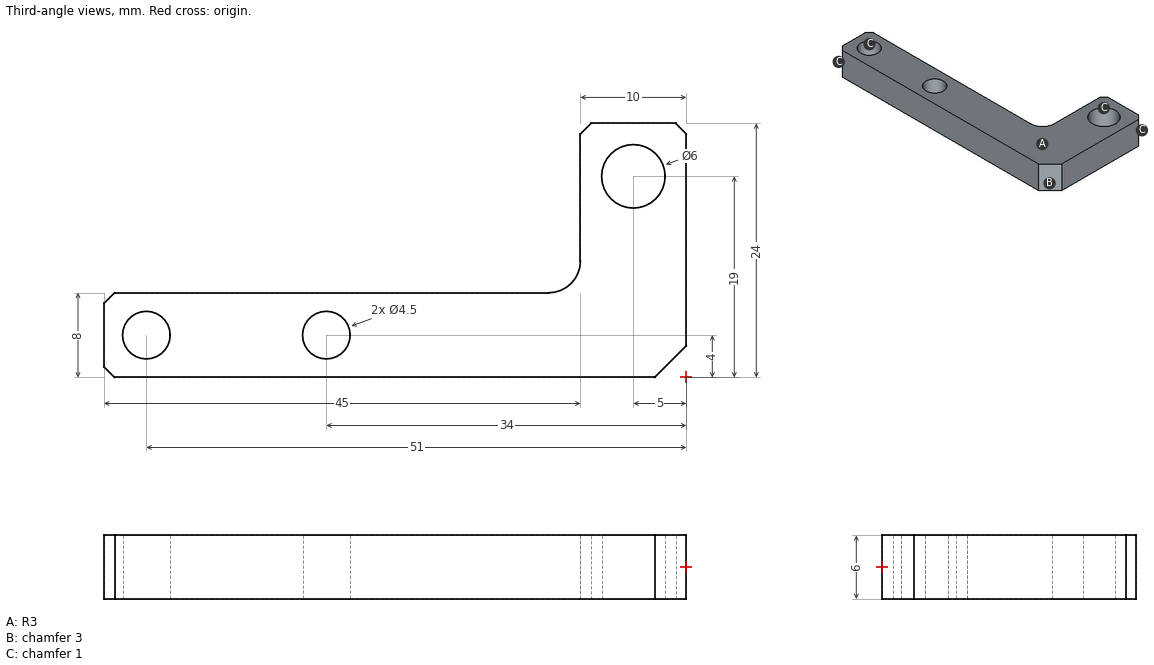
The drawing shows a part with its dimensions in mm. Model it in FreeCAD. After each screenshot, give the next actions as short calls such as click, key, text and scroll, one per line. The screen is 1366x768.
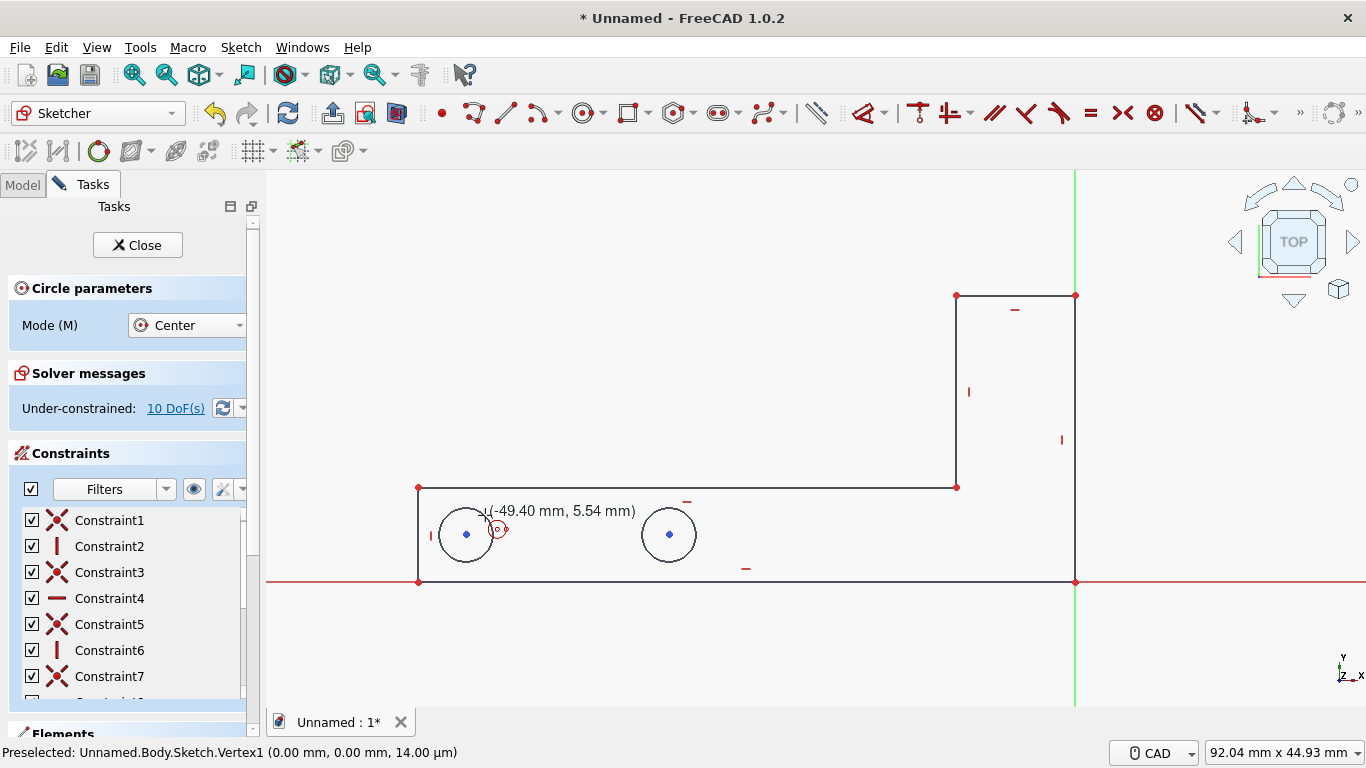
click(1016, 355)
click(1041, 330)
key(Escape)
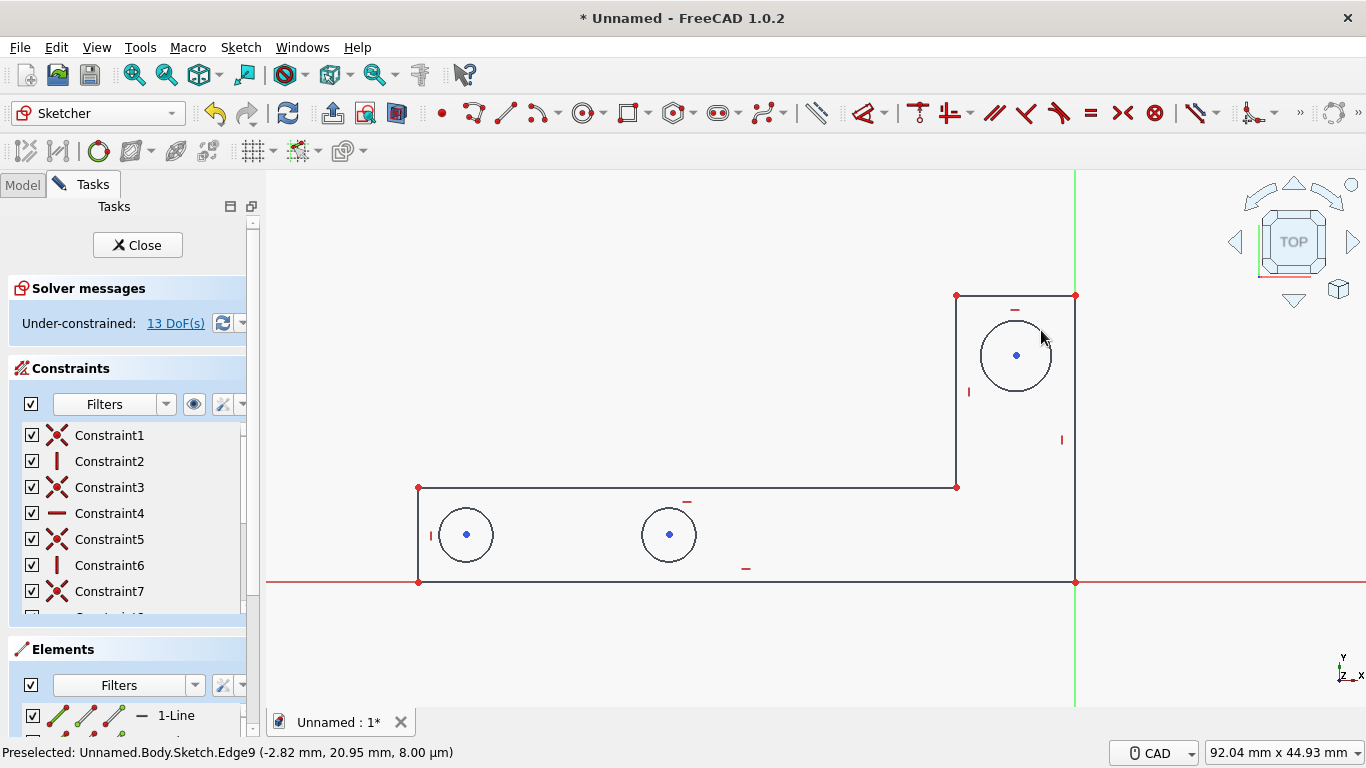
click(688, 516)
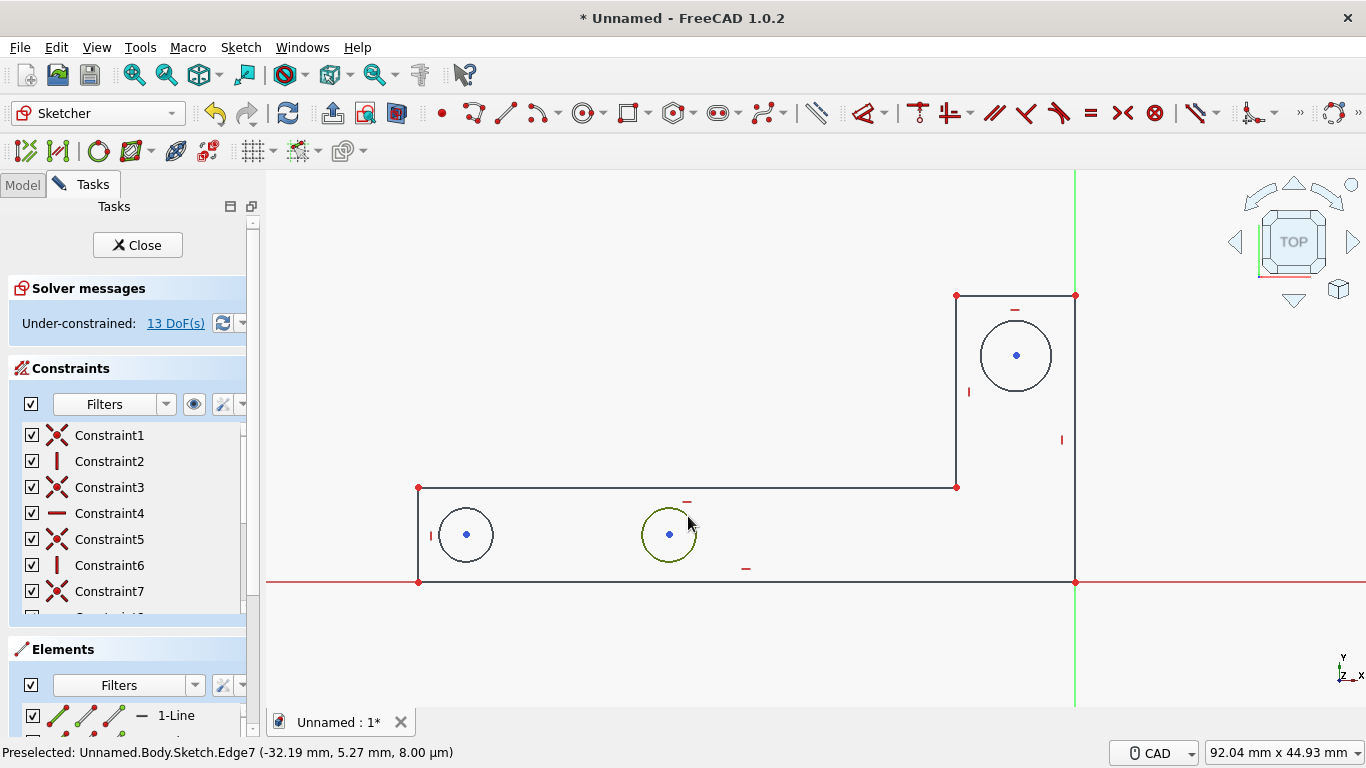
click(485, 516)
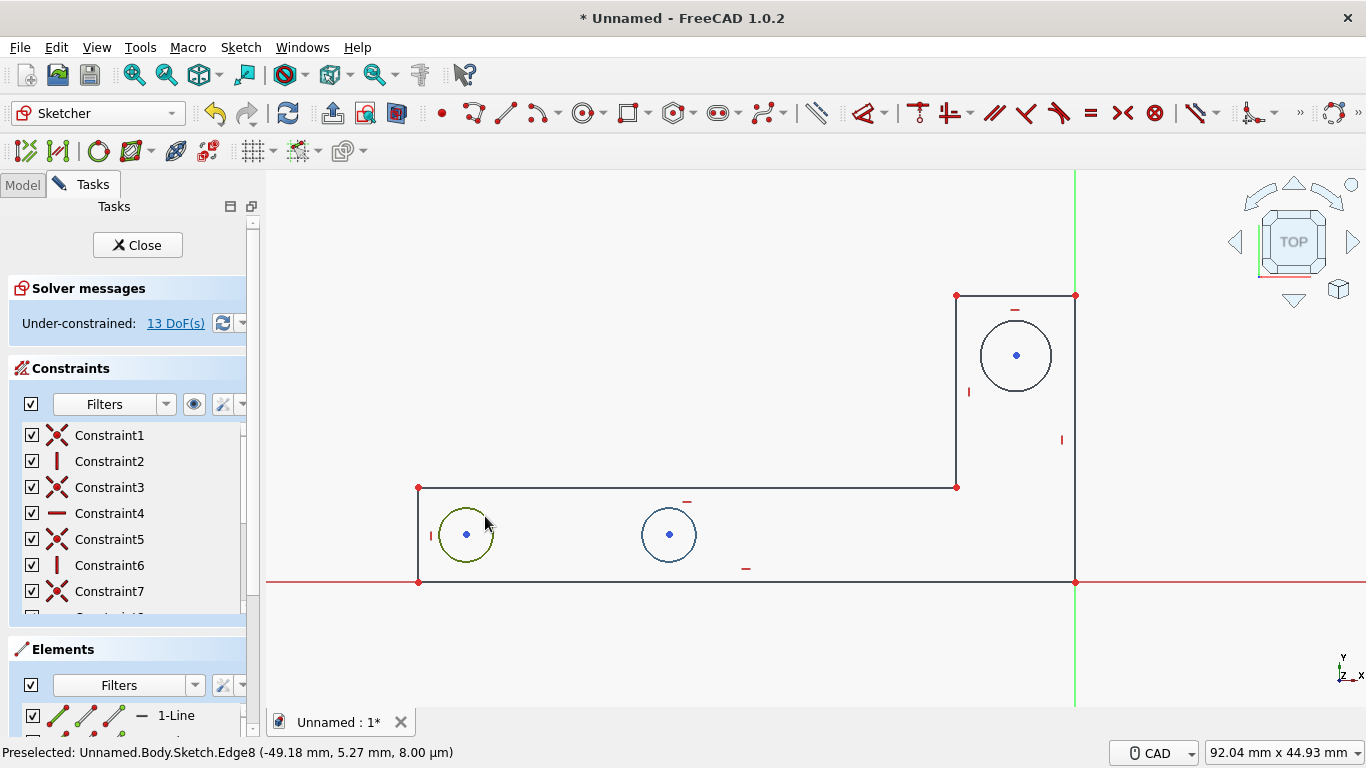
click(1092, 114)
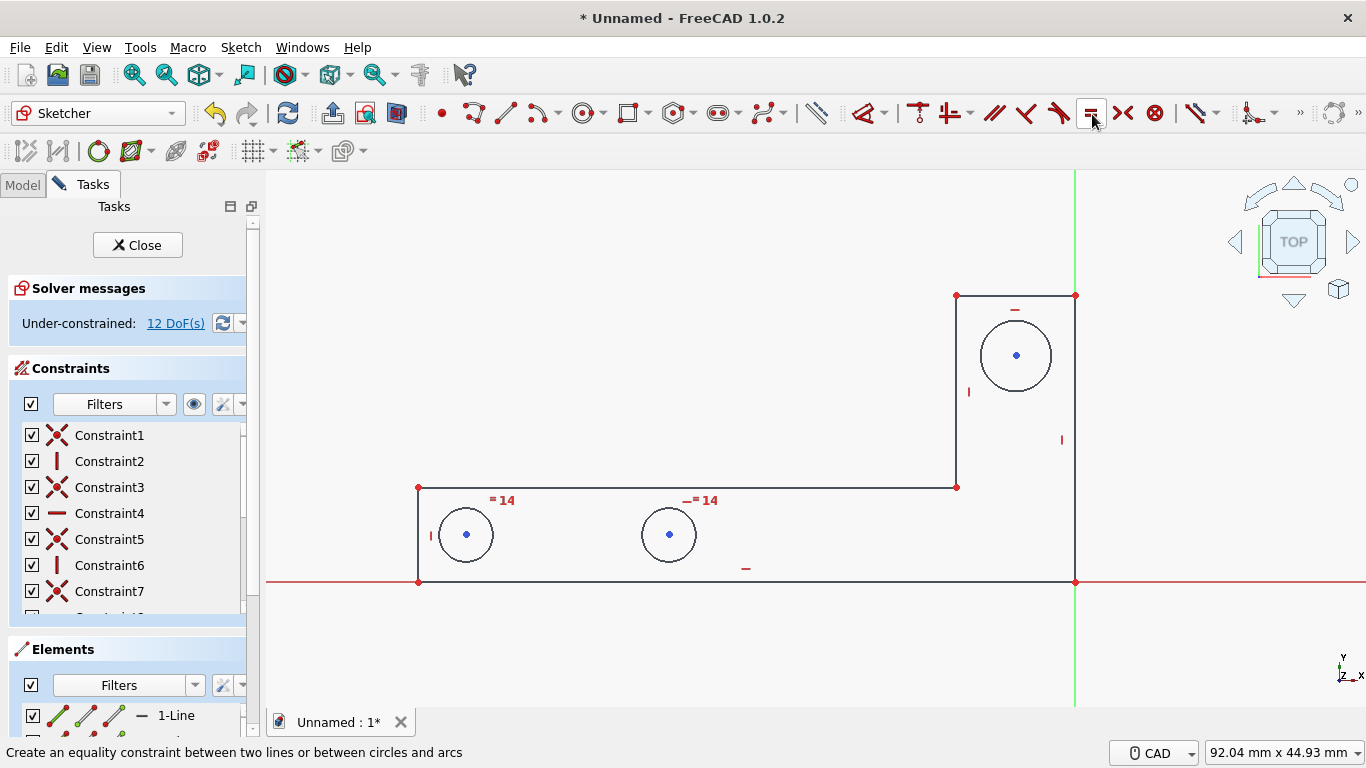
click(669, 535)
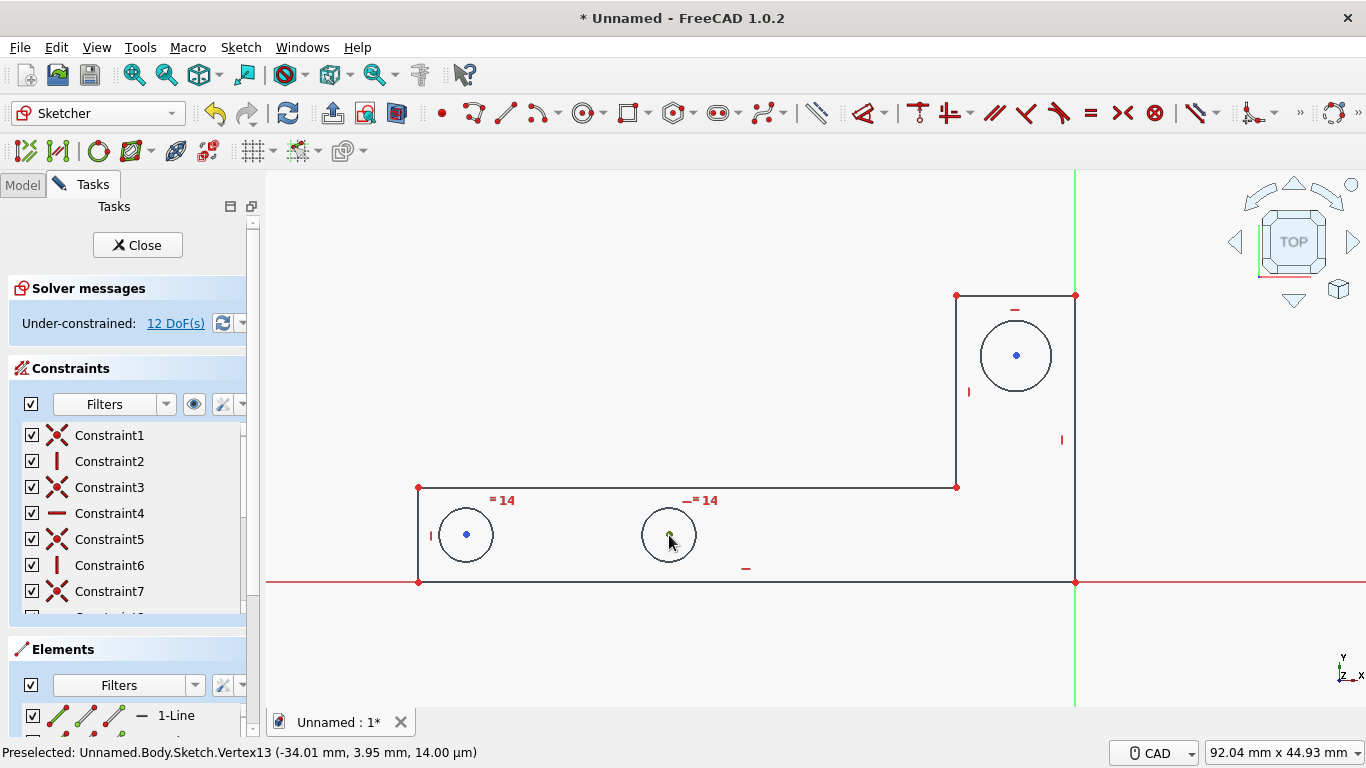
click(466, 535)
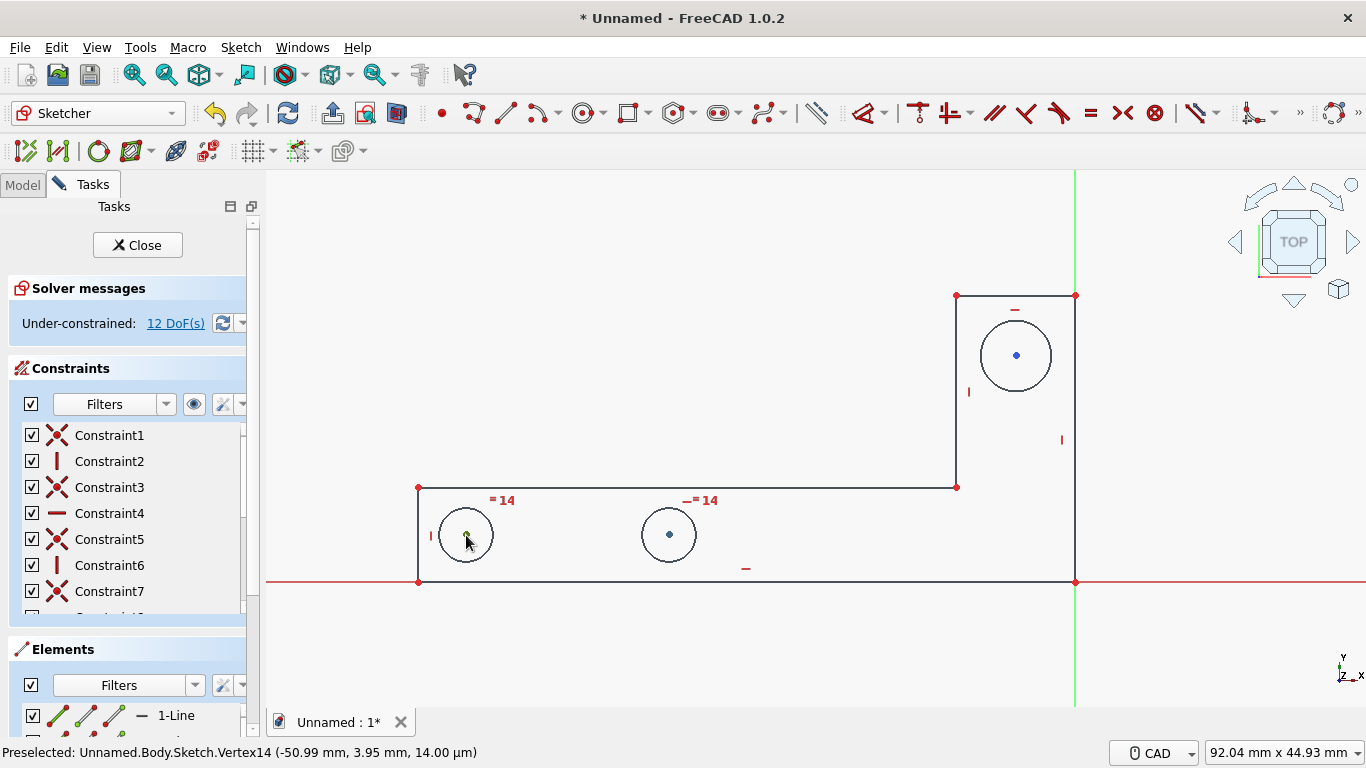
key(h)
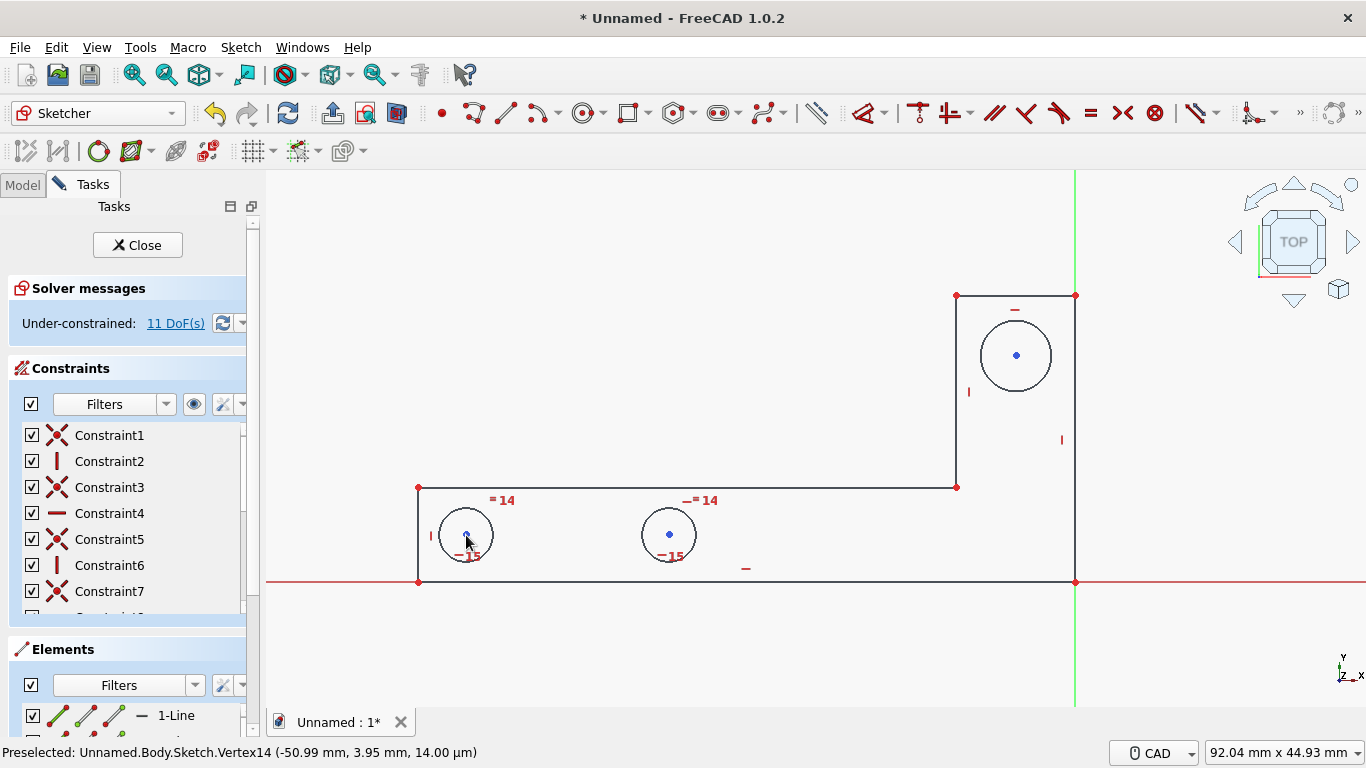
click(688, 516)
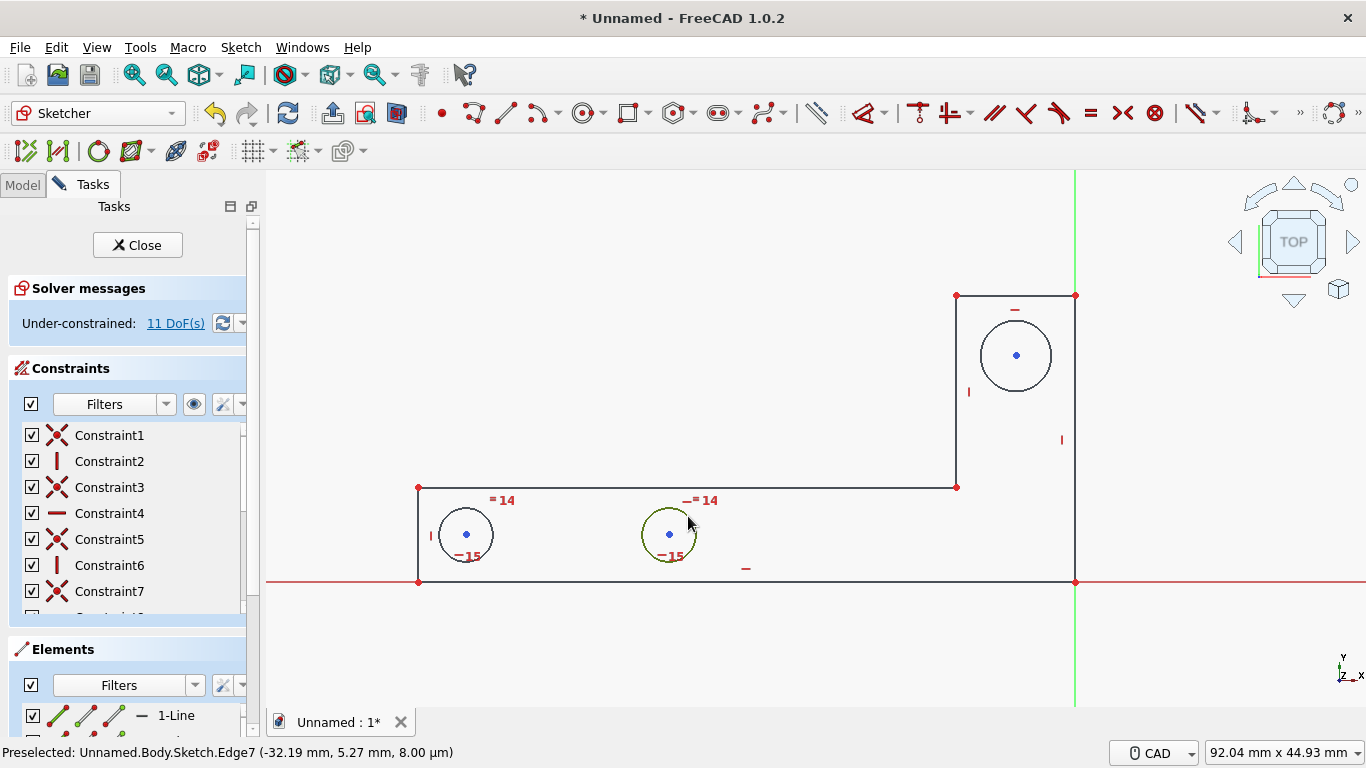
click(886, 114)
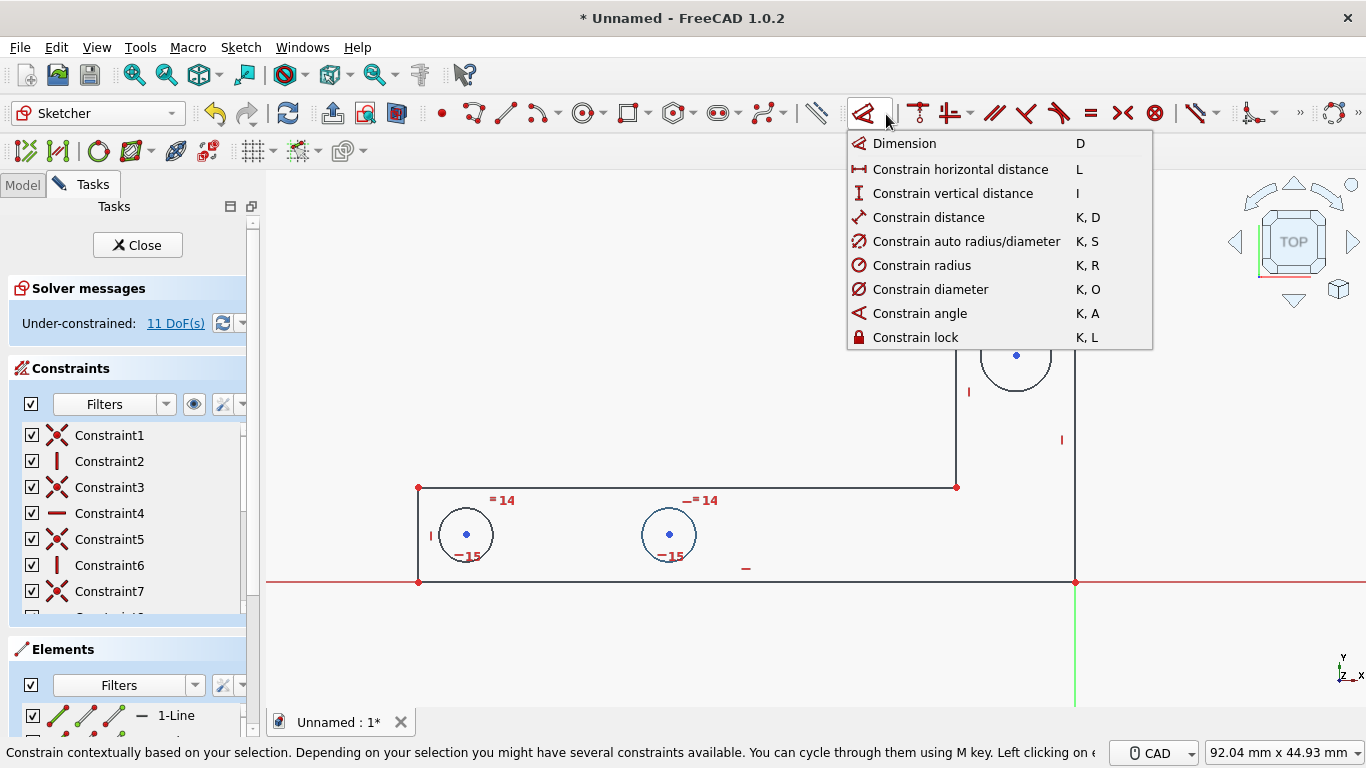
click(1000, 289)